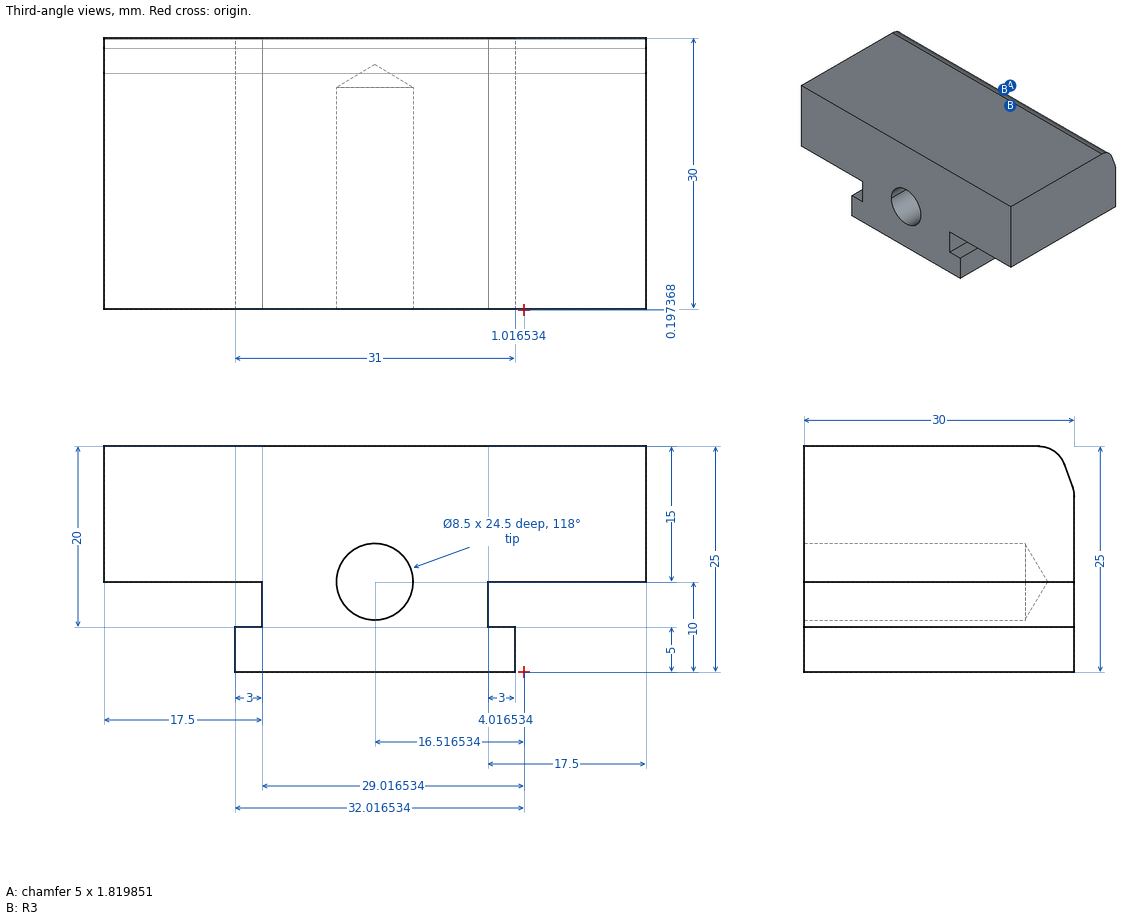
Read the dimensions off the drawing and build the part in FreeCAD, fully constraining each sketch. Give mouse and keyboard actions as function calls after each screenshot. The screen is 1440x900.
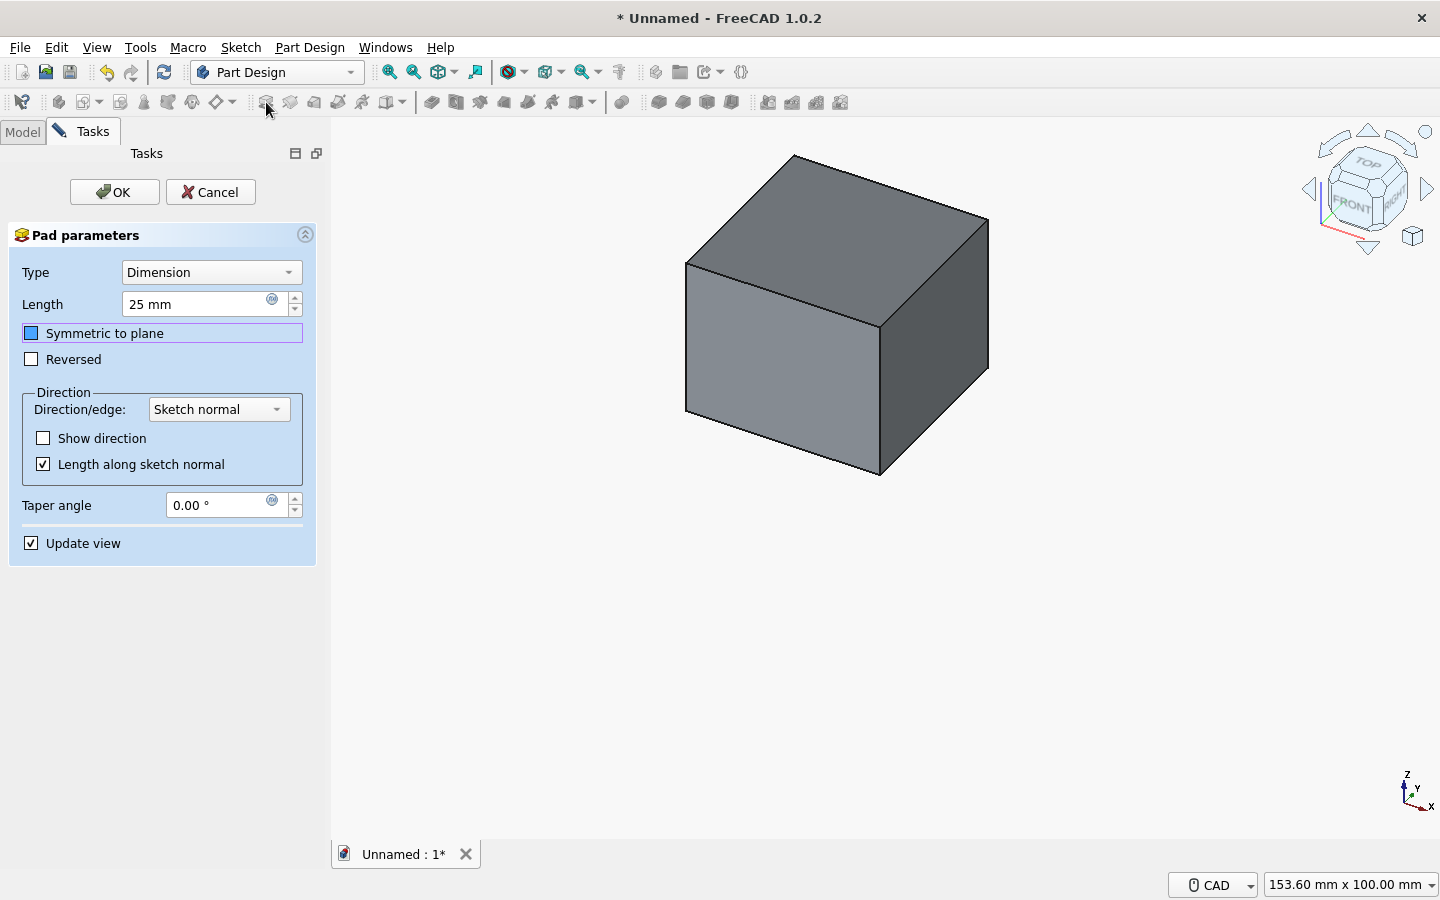
click(115, 192)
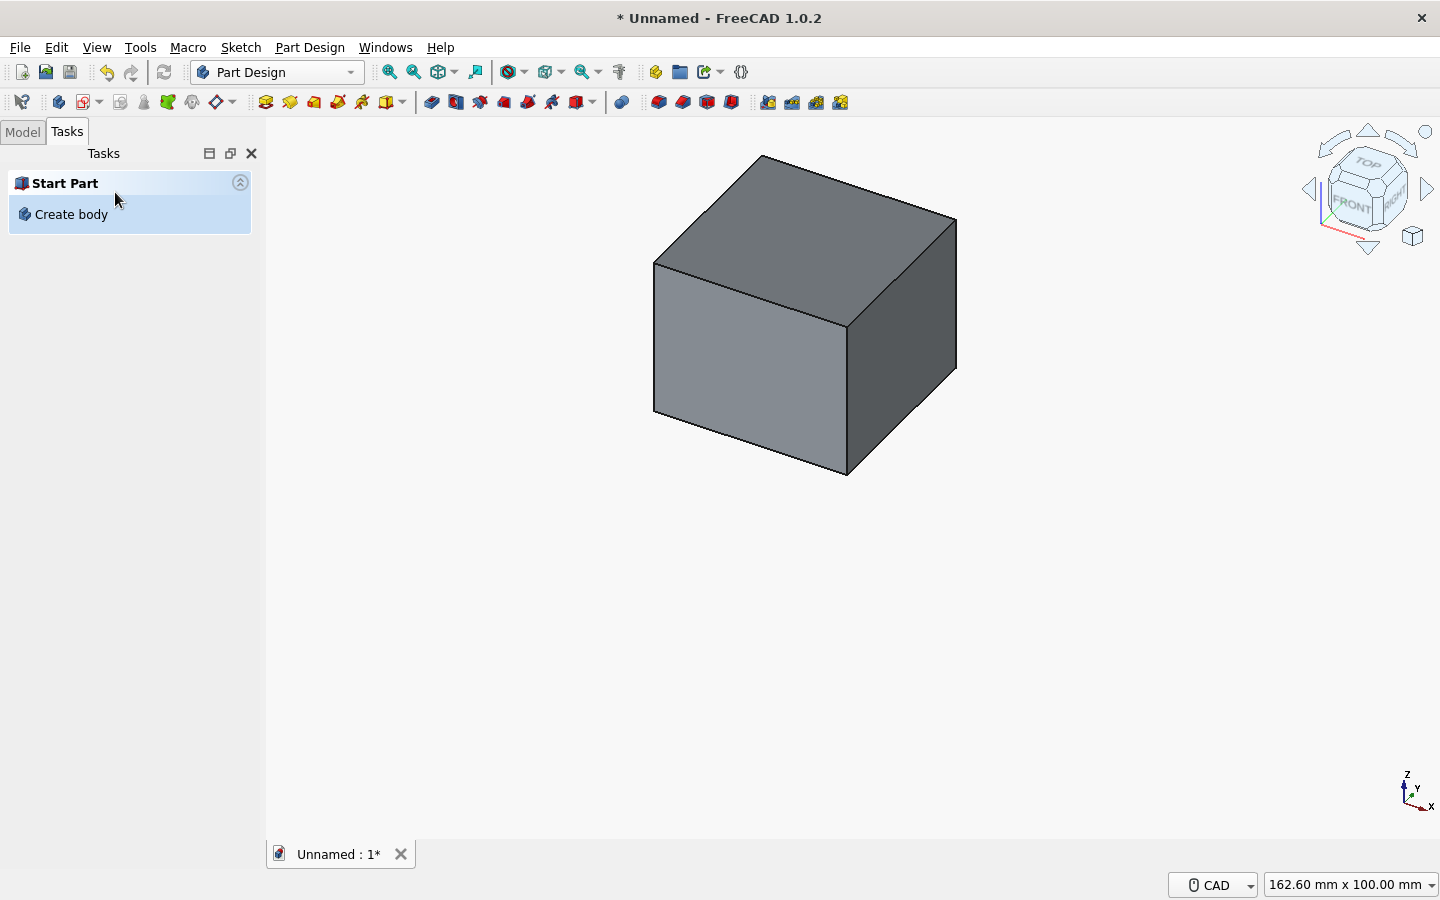
click(390, 72)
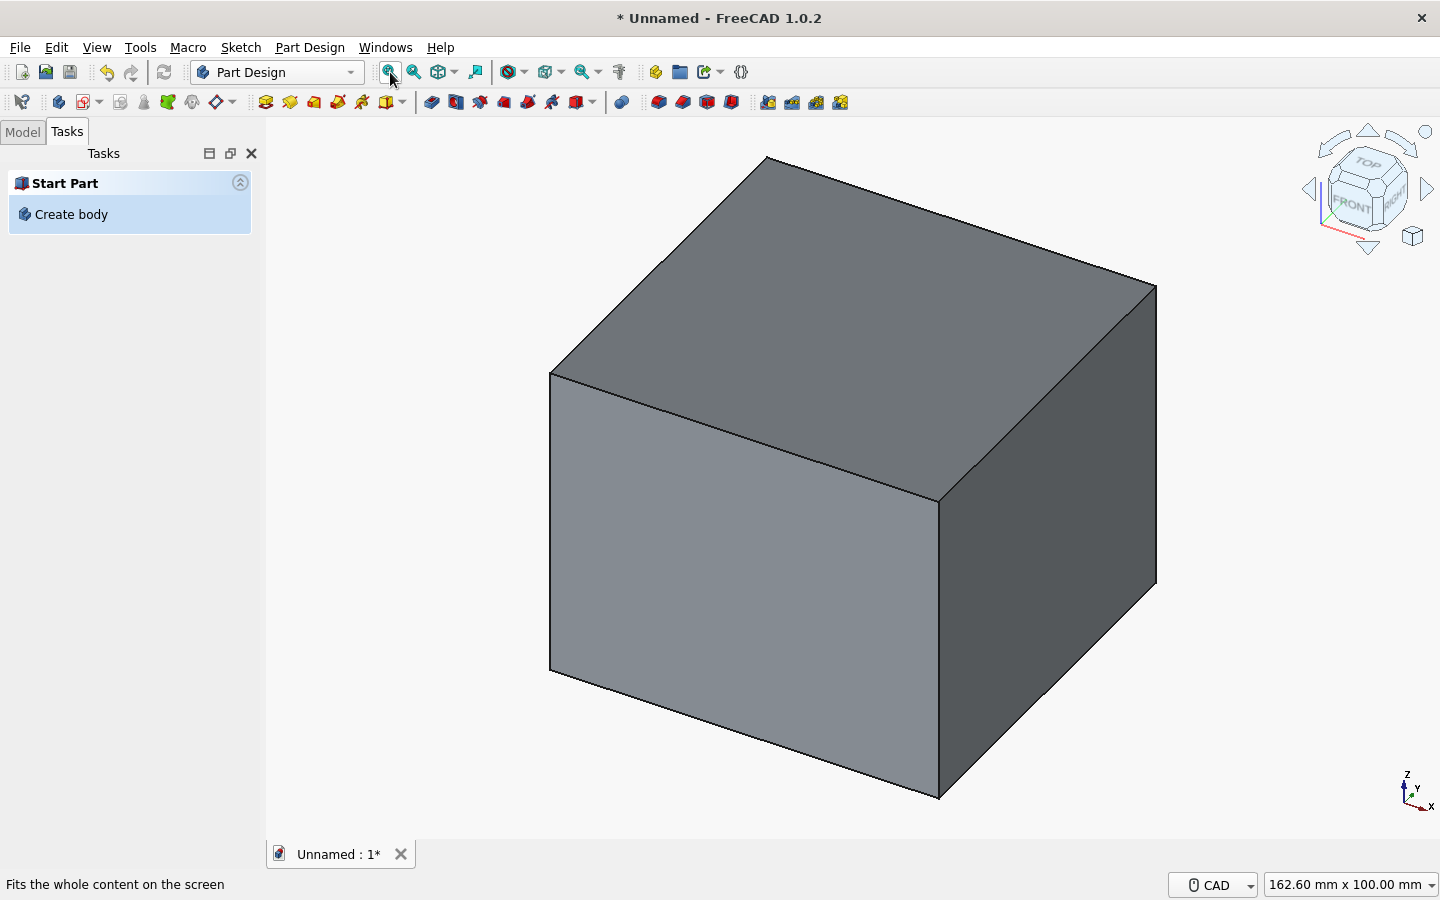
click(744, 585)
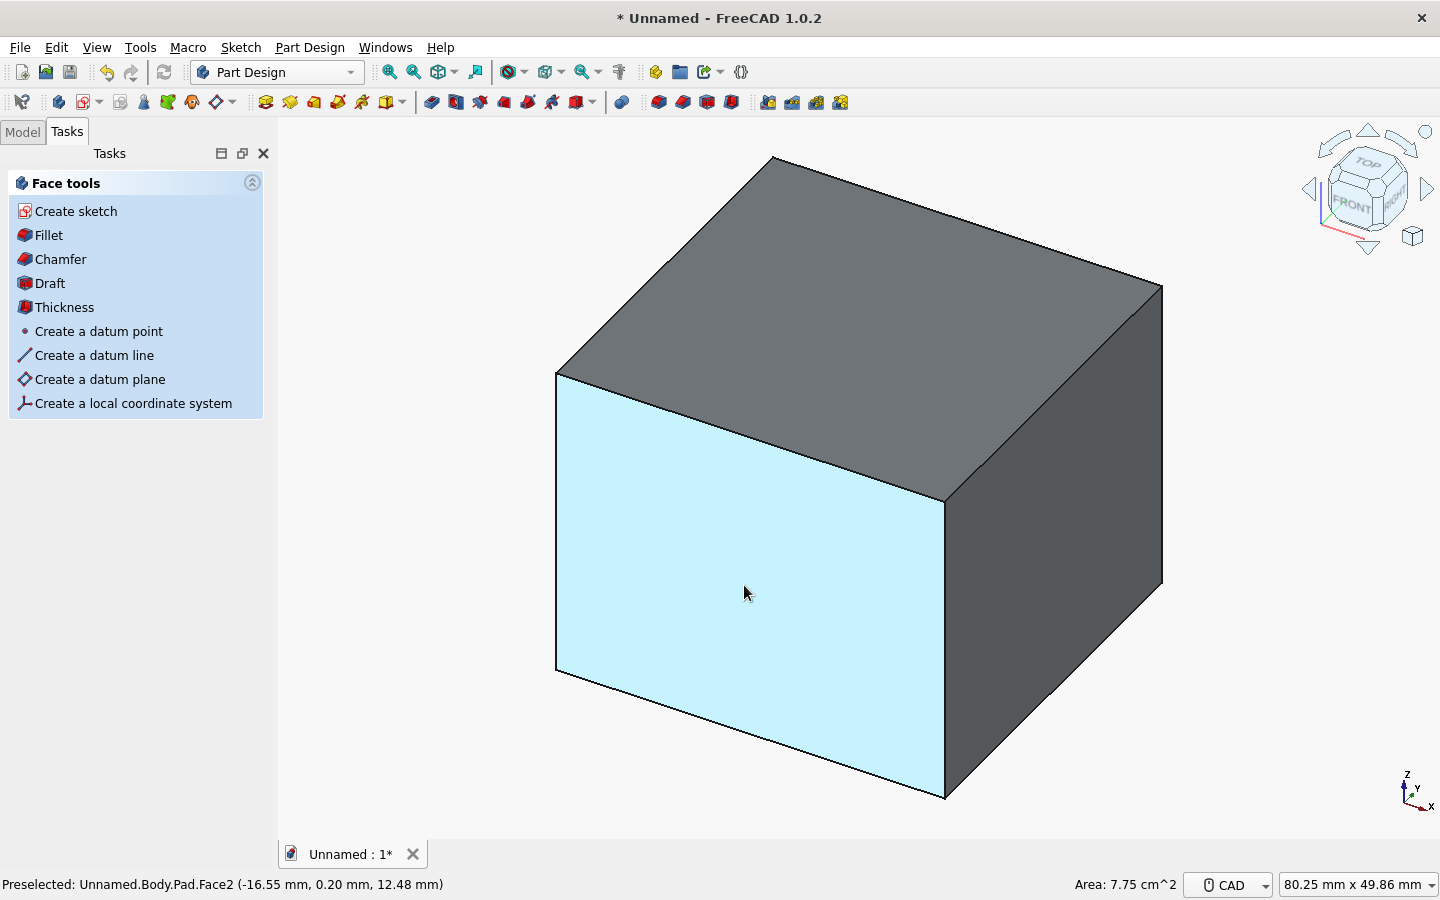
click(84, 102)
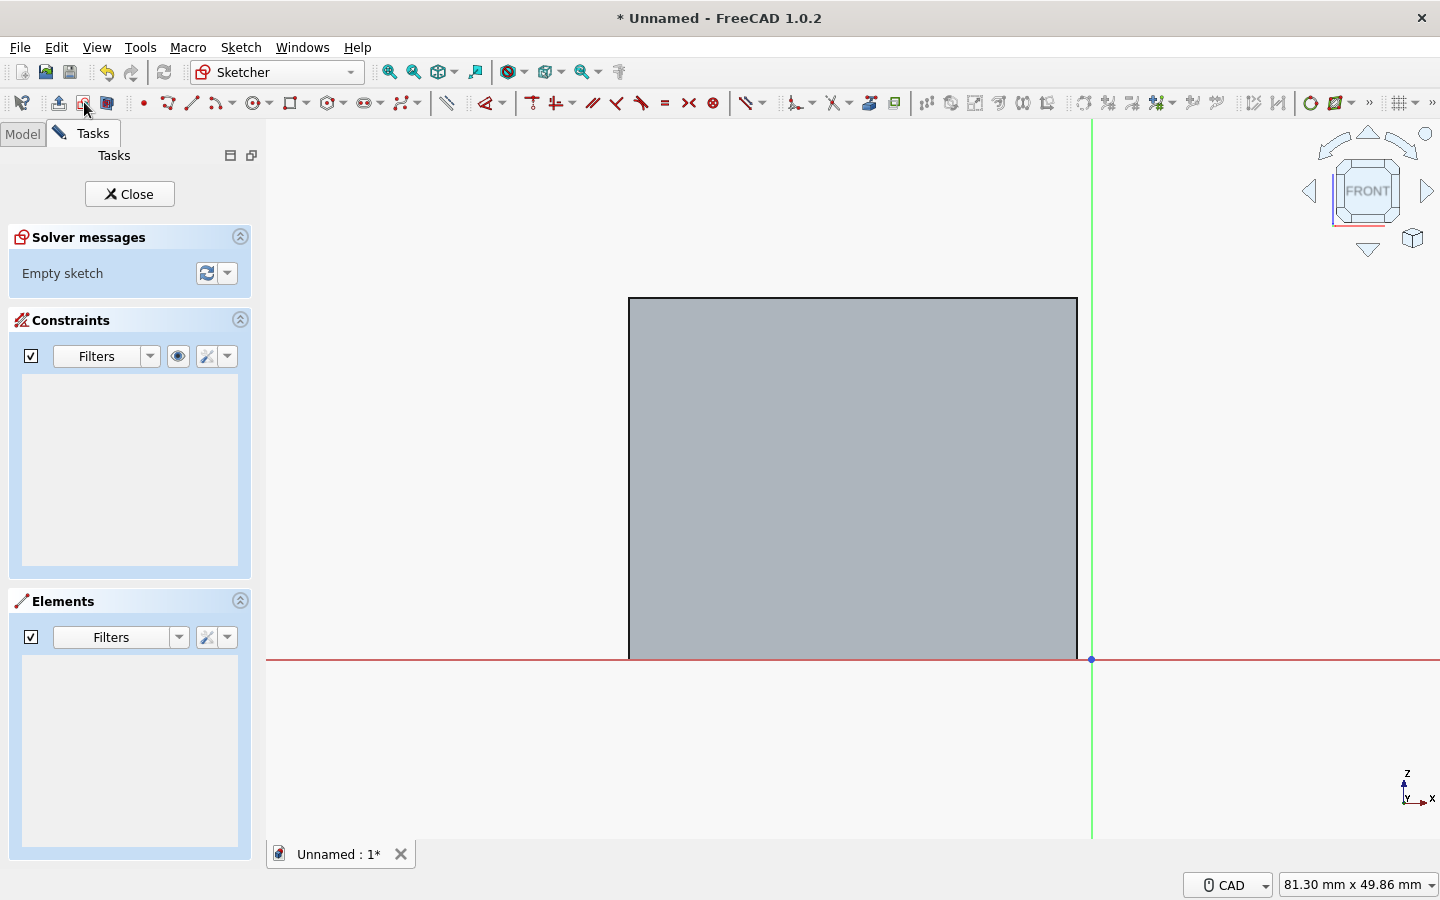
click(290, 104)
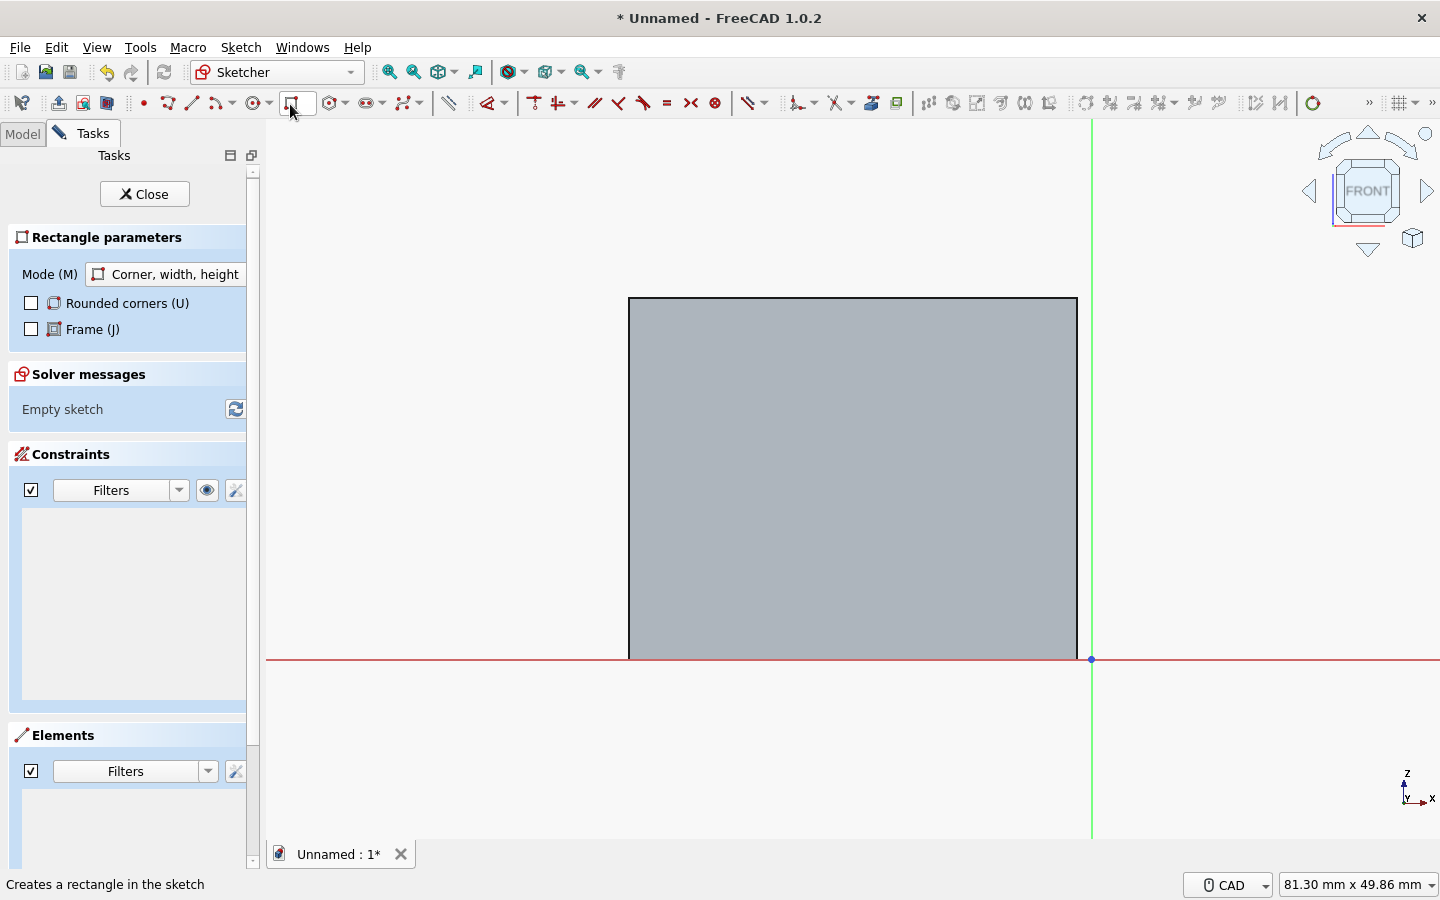
click(629, 298)
move(672, 587)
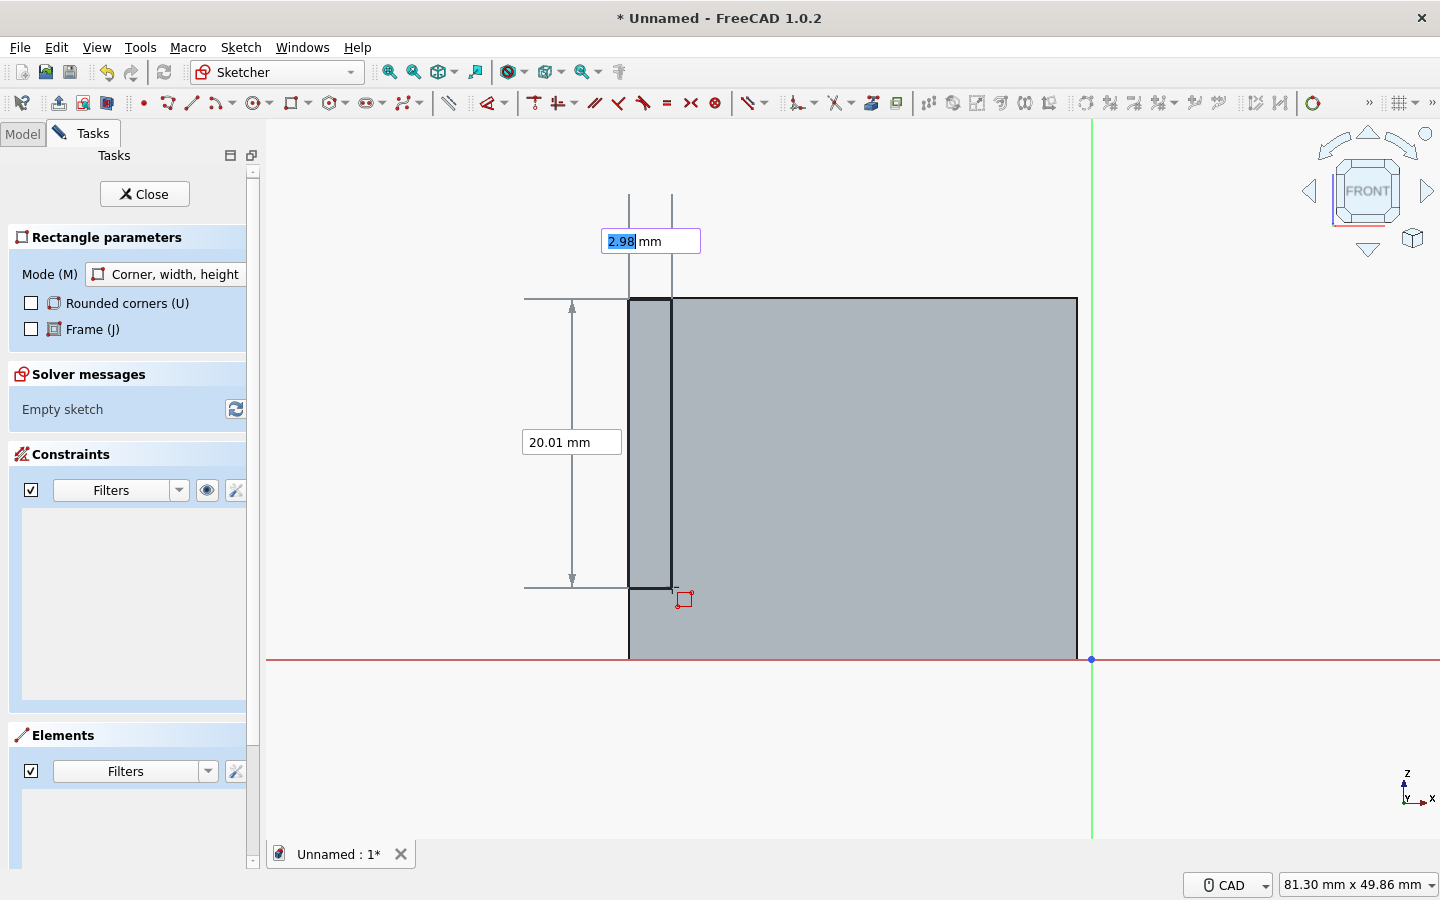
text(3)
key(Tab)
text(20)
key(Return)